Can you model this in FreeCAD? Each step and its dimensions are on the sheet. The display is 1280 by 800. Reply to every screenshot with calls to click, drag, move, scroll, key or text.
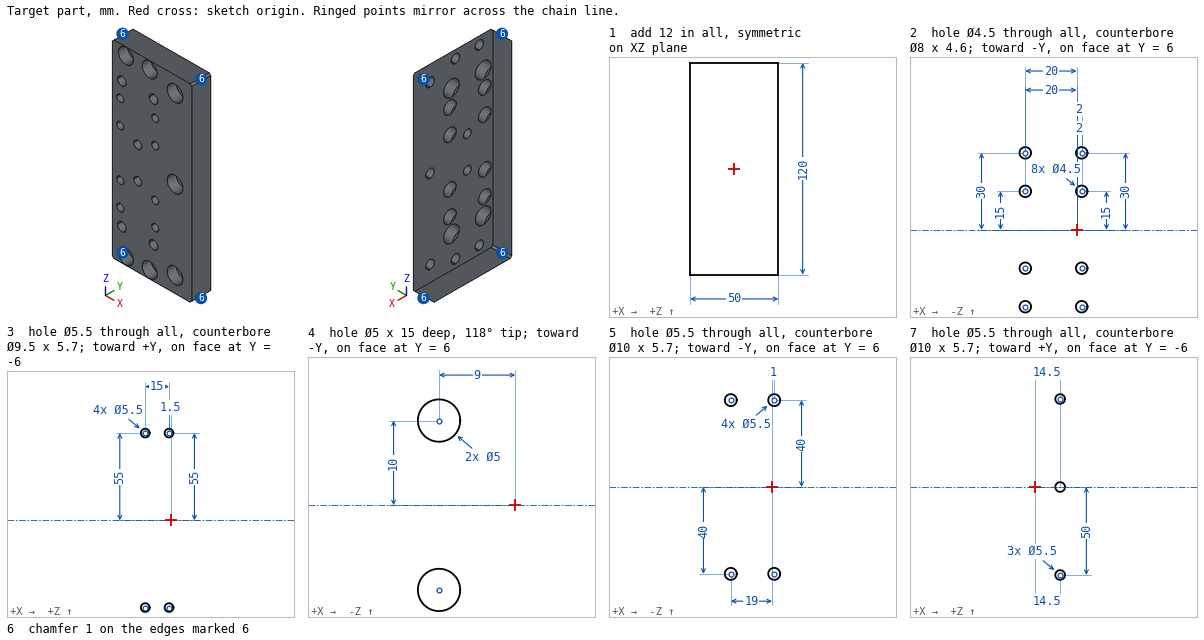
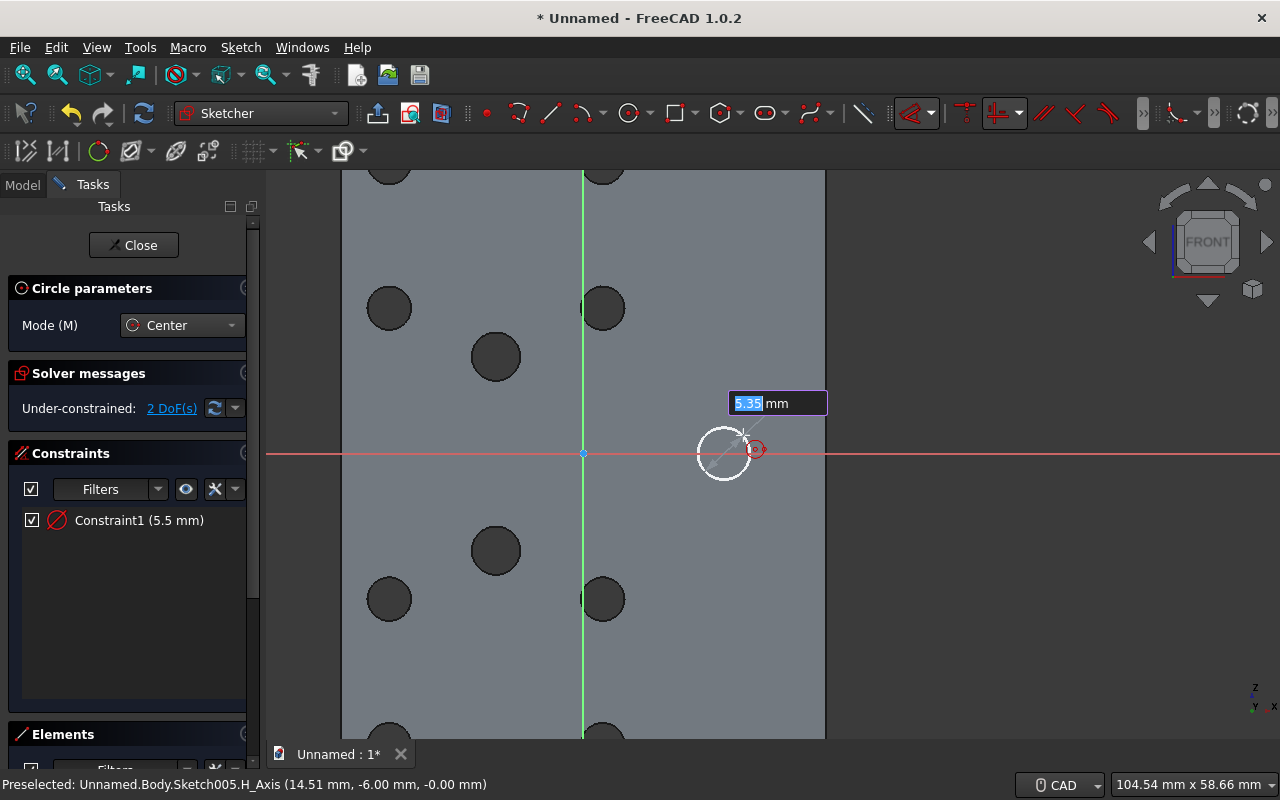
text(5.5)
key(Return)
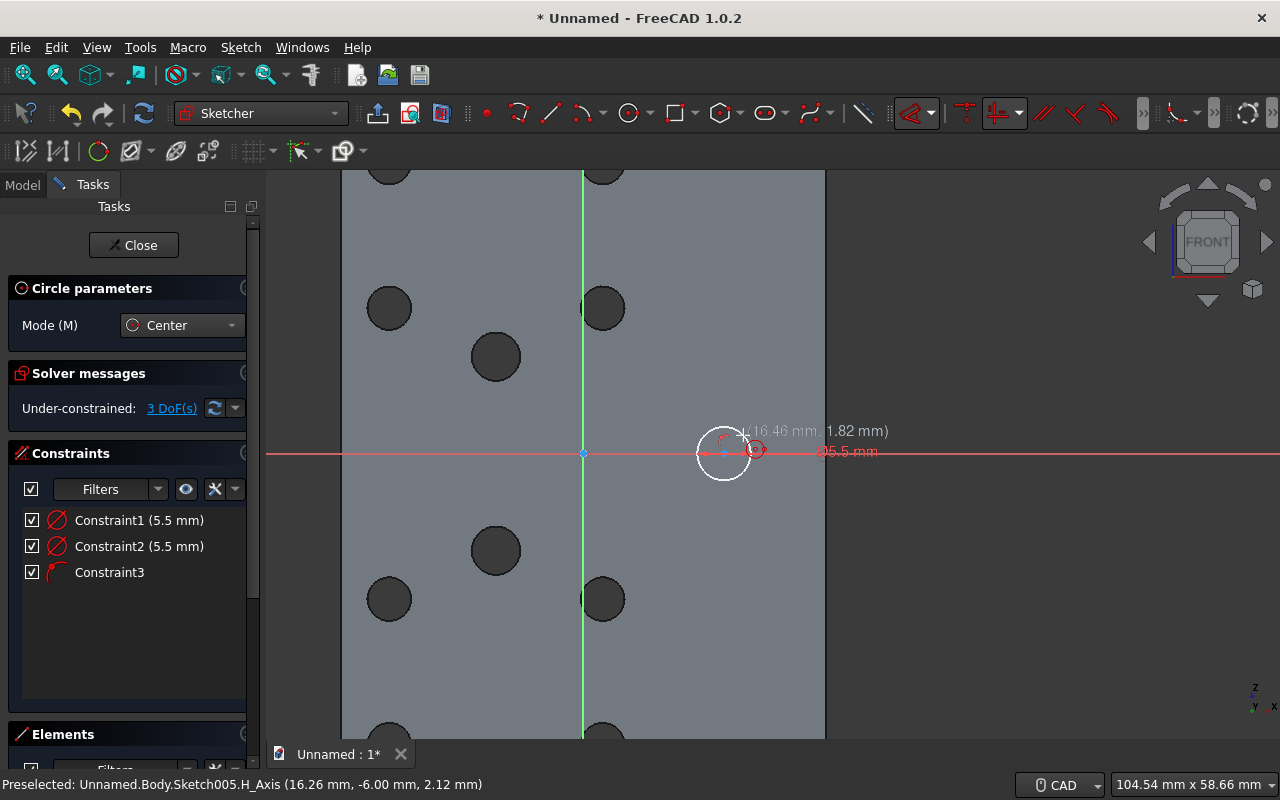
scroll(726, 455, down, 5)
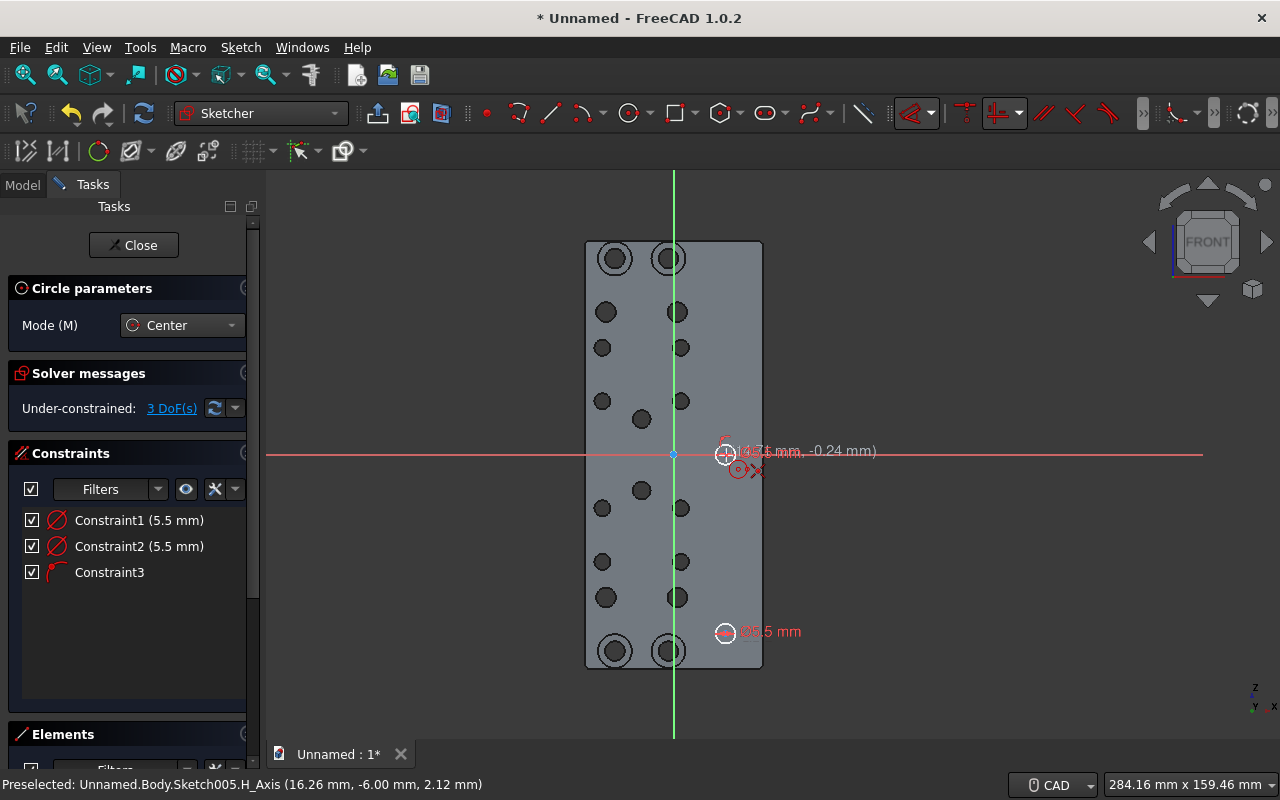
scroll(726, 276, up, 5)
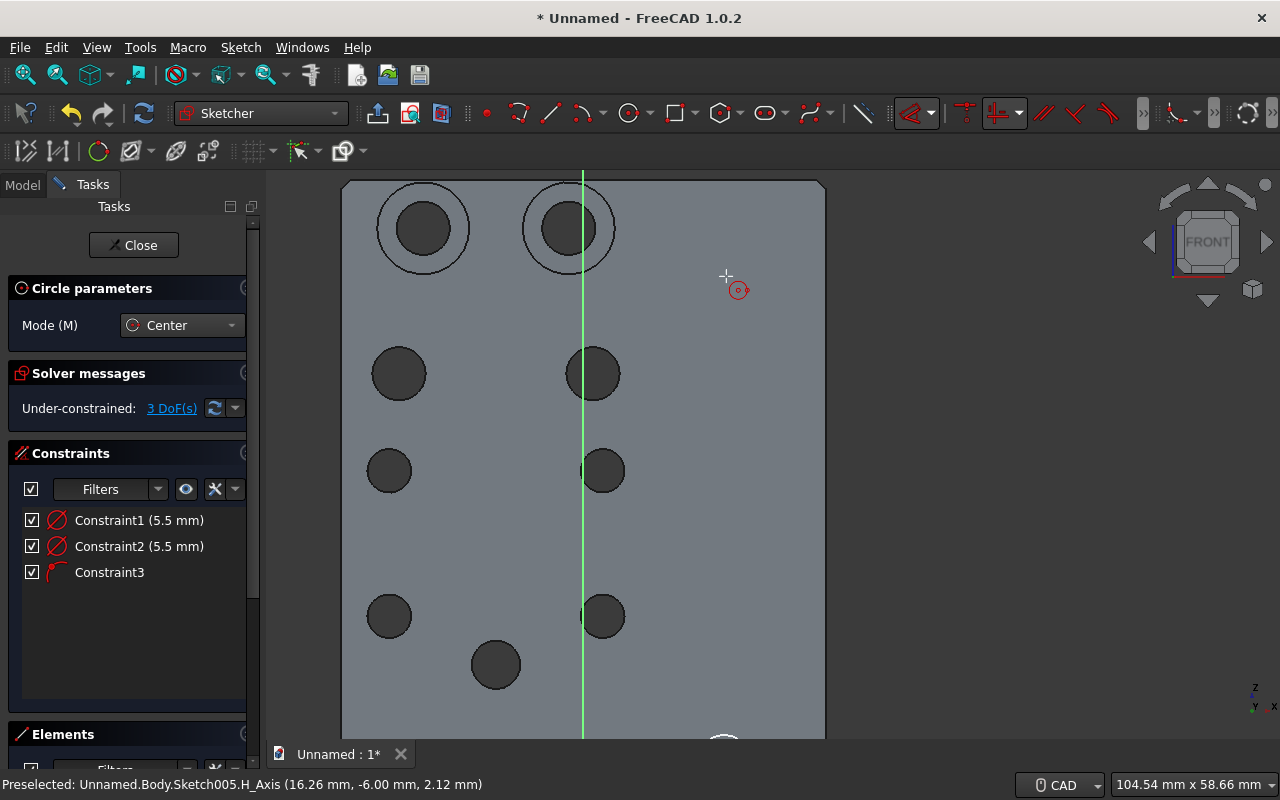
click(724, 277)
move(743, 258)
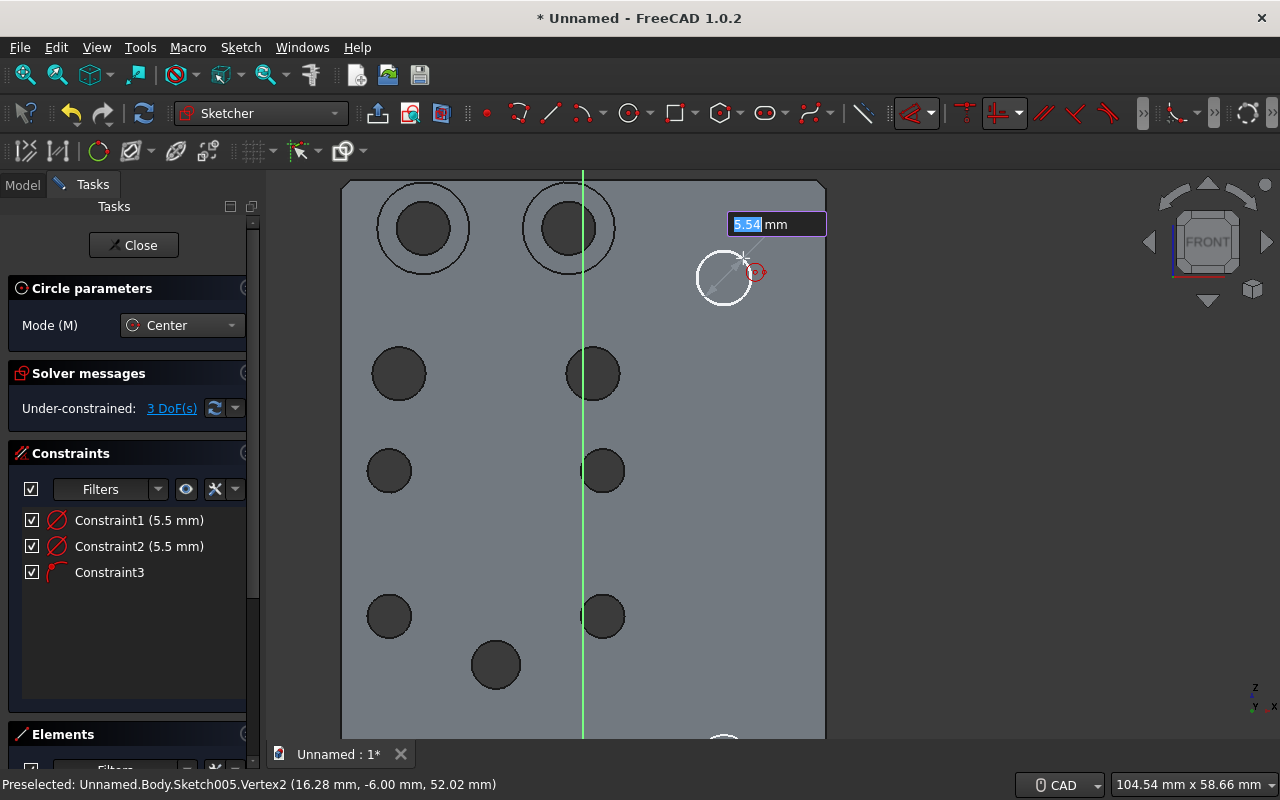
text(5.5)
key(Return)
key(Escape)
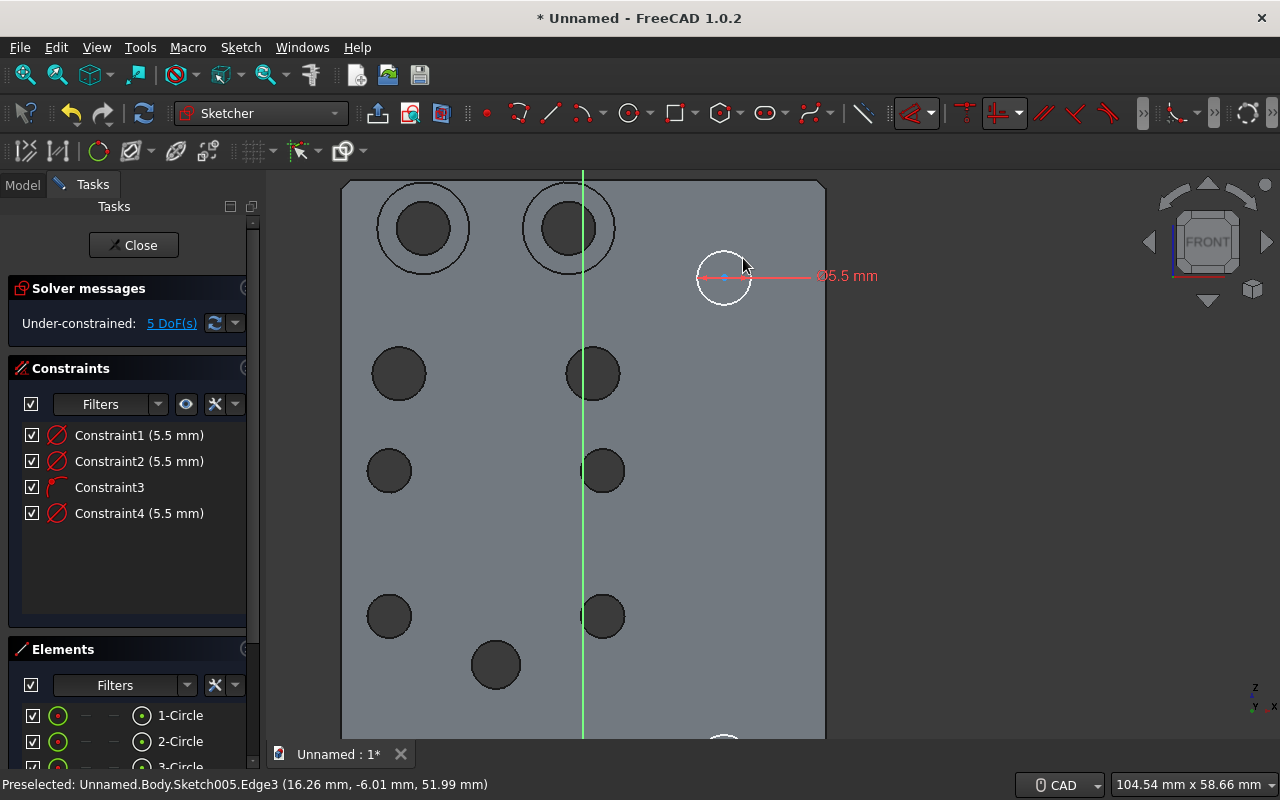
scroll(726, 276, down, 5)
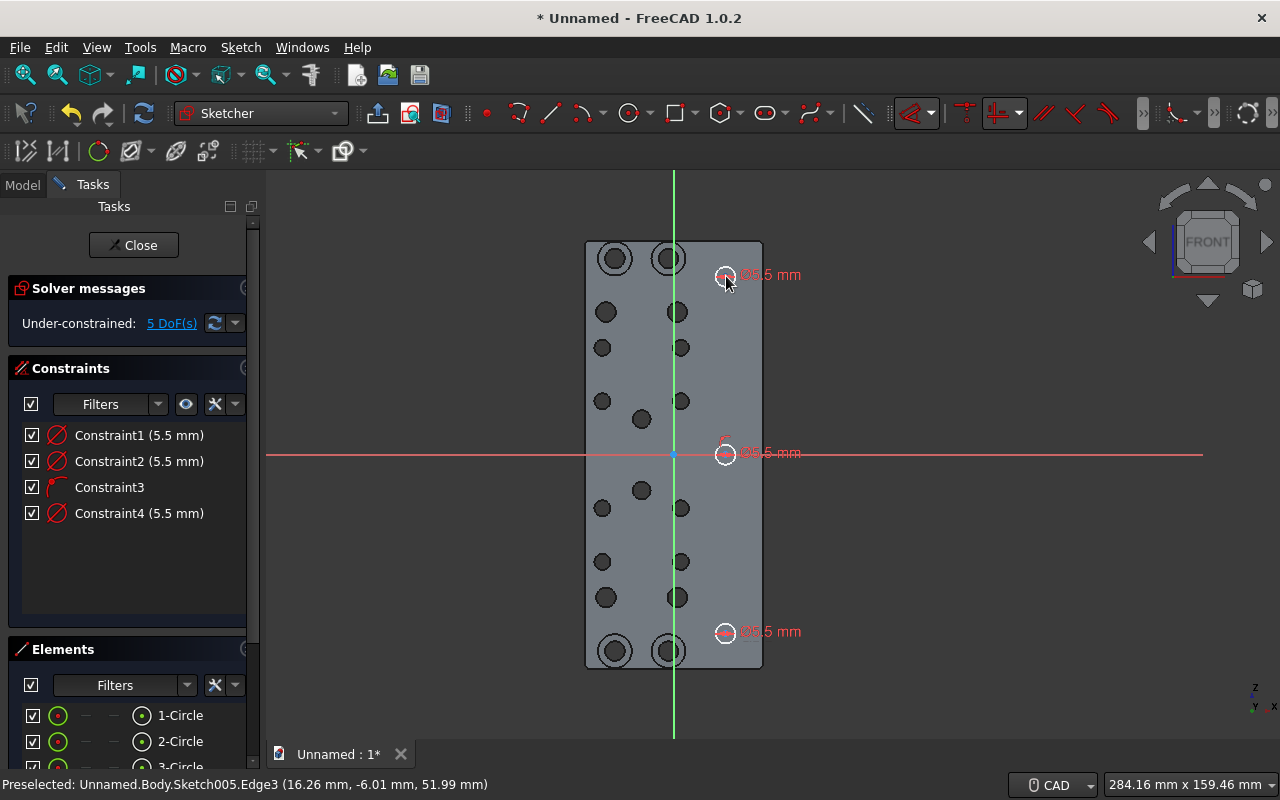
click(726, 634)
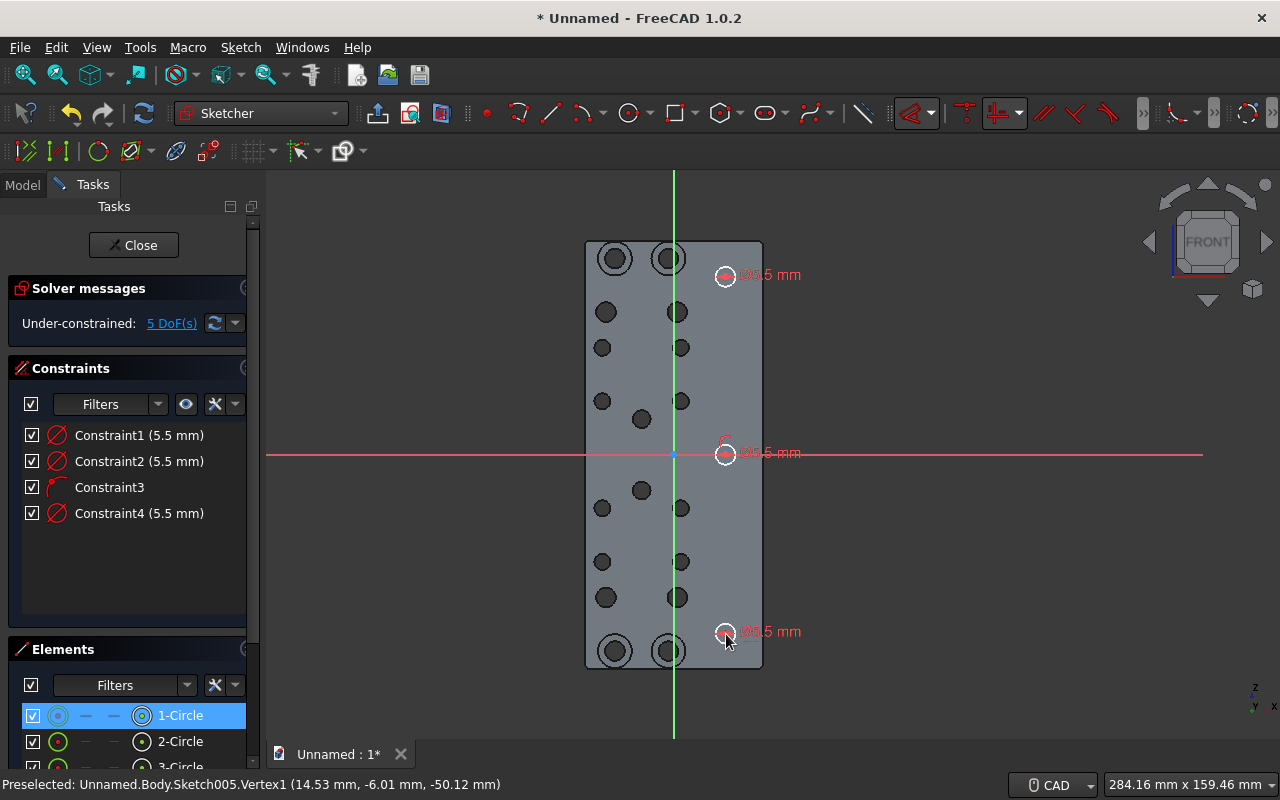
click(726, 277)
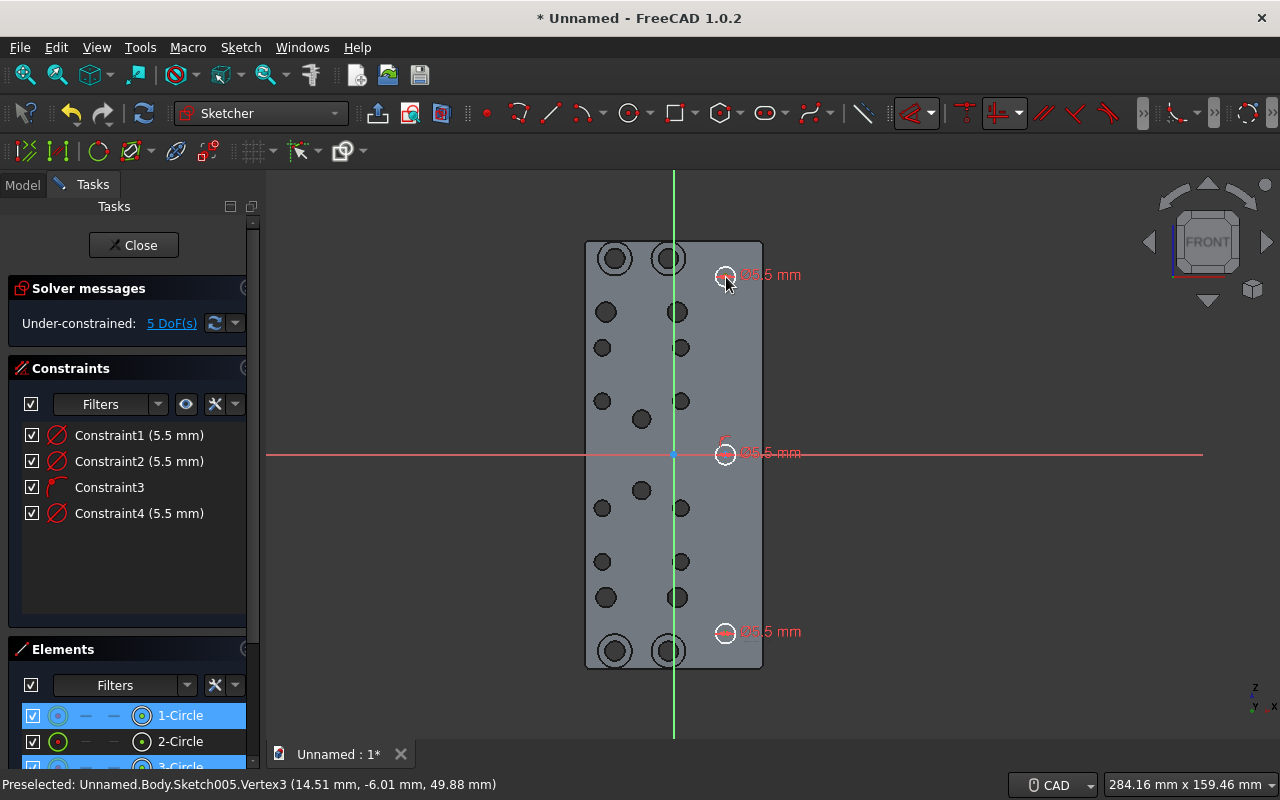
click(353, 455)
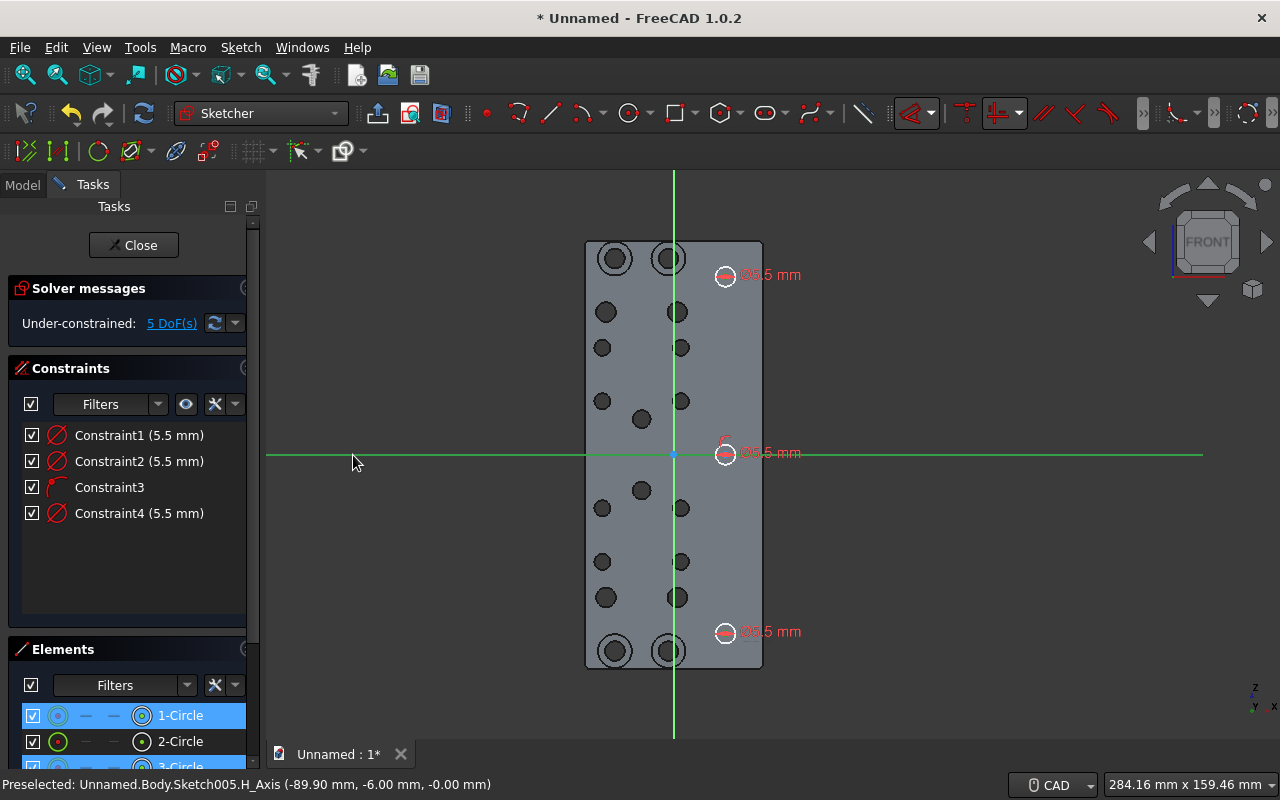
key(s)